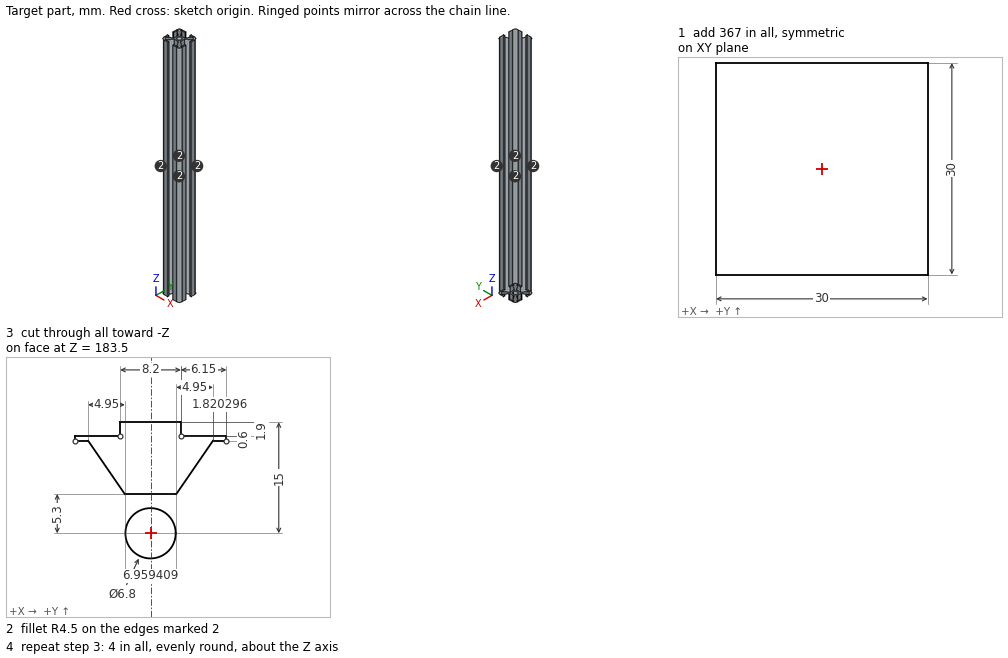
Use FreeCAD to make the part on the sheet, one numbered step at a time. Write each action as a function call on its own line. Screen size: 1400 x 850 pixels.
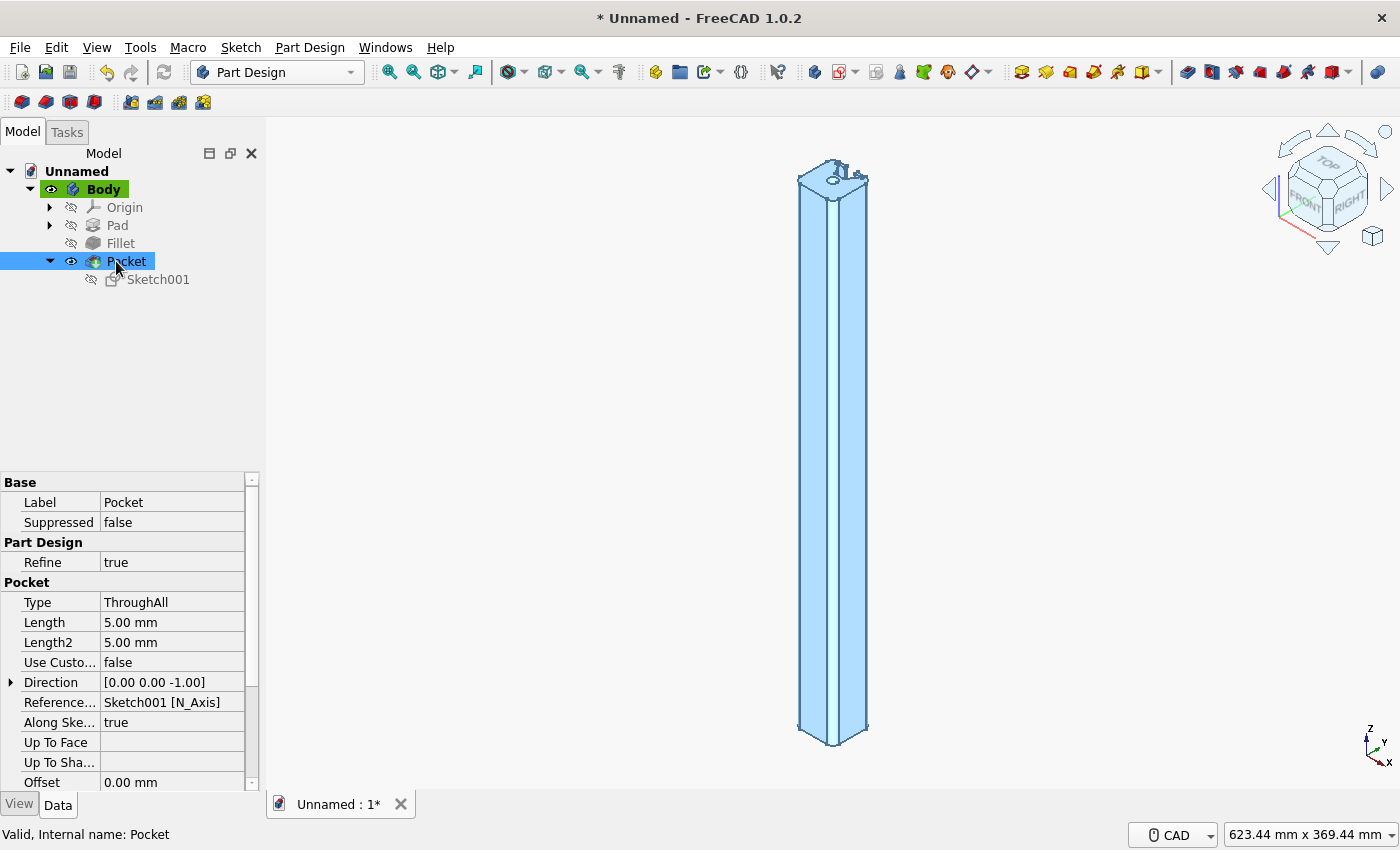
click(180, 102)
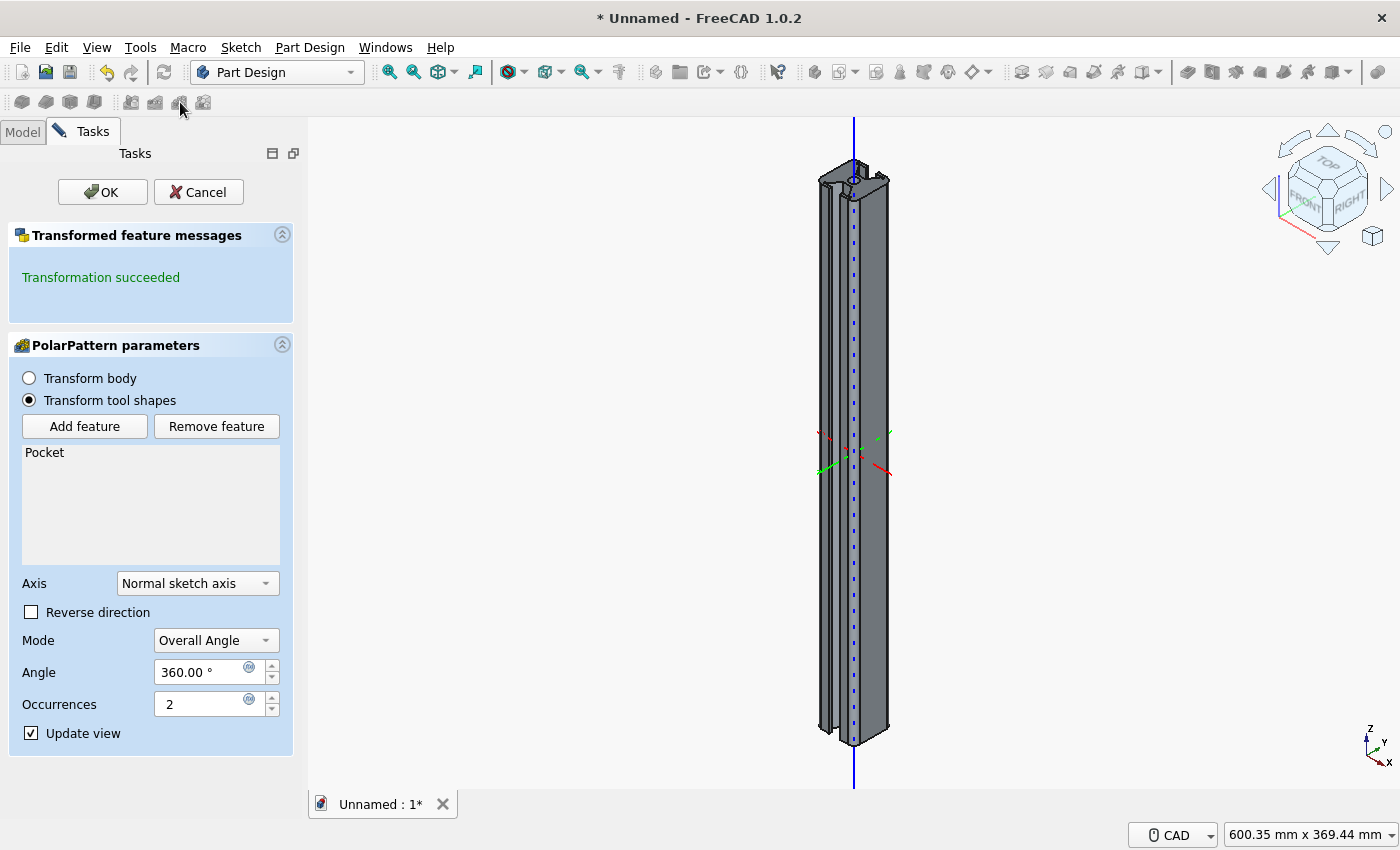
click(198, 584)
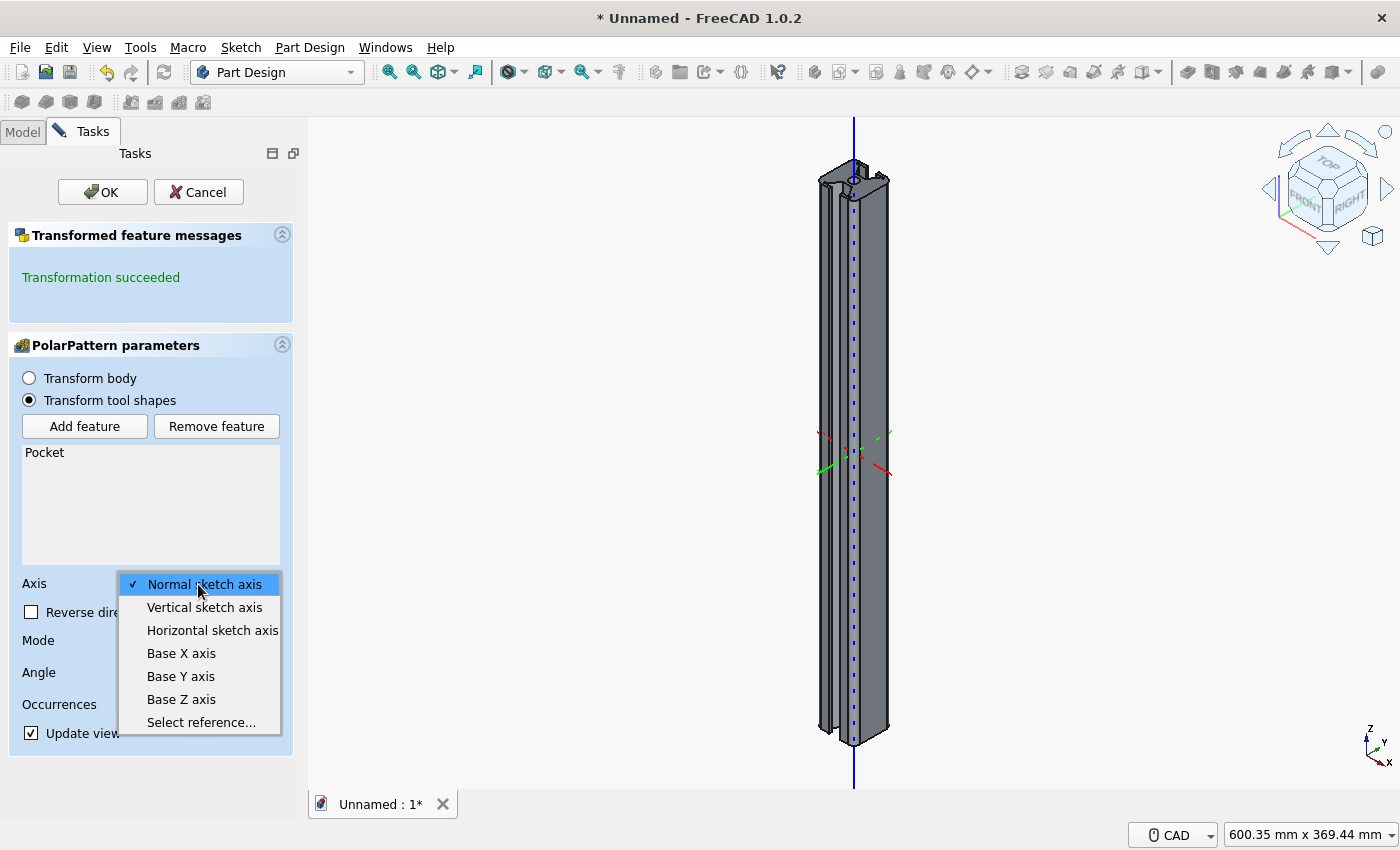
click(198, 700)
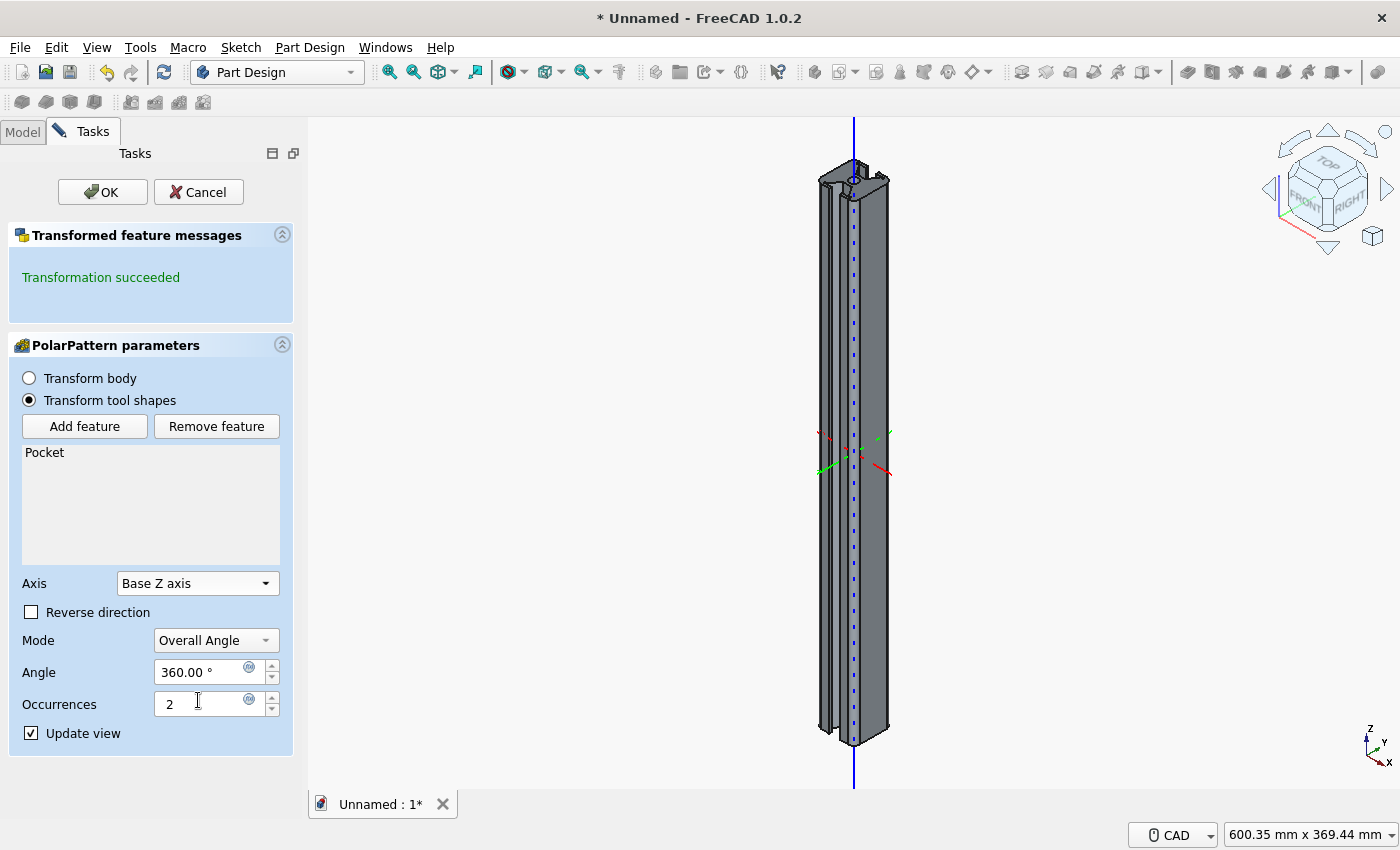
triple_click(209, 704)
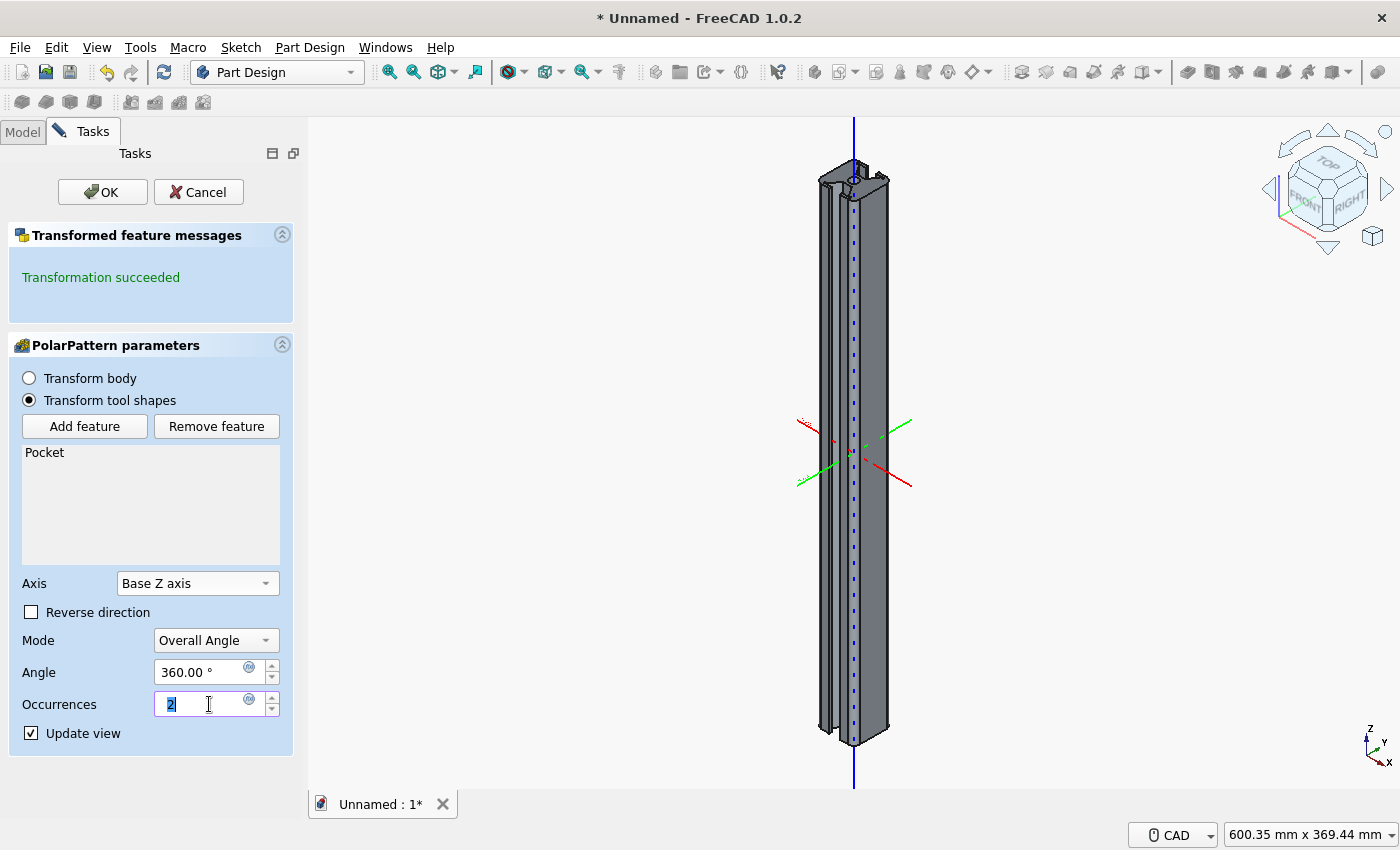
text(4)
key(Tab)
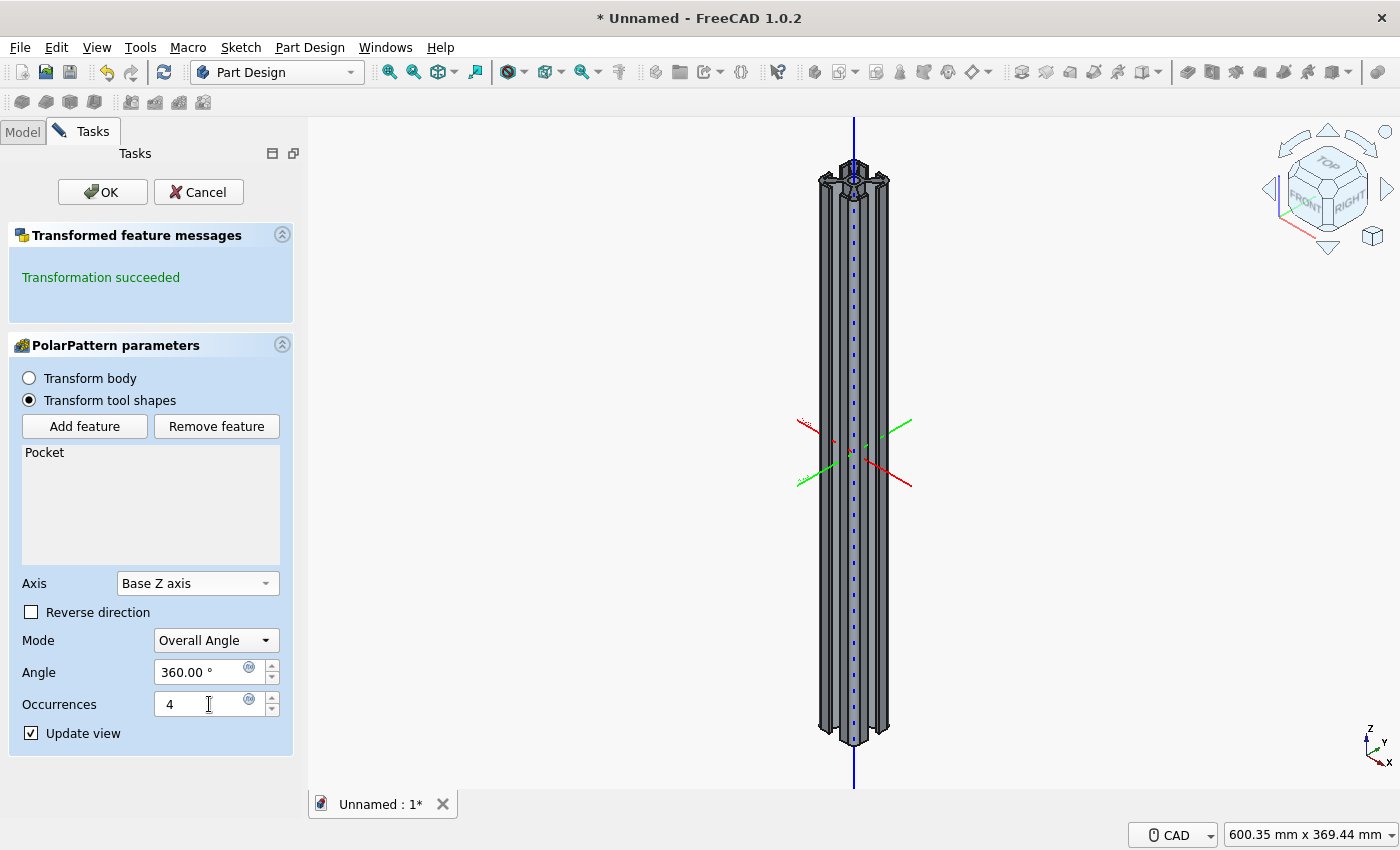
click(103, 192)